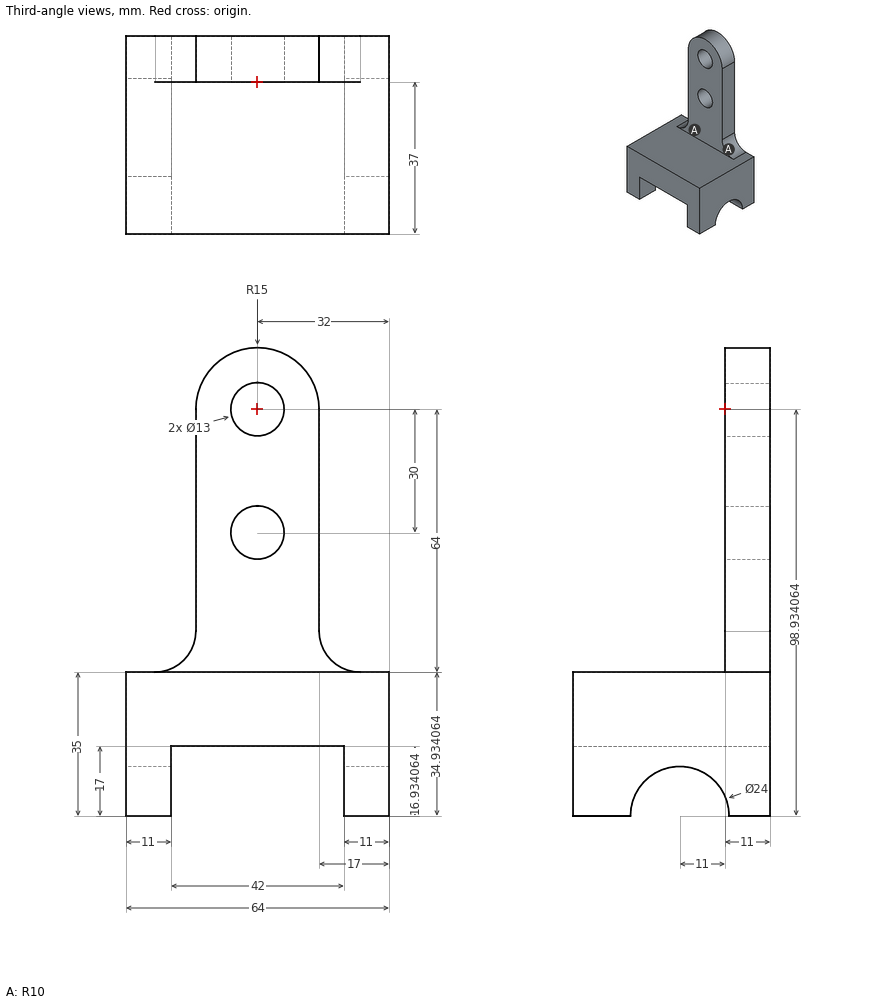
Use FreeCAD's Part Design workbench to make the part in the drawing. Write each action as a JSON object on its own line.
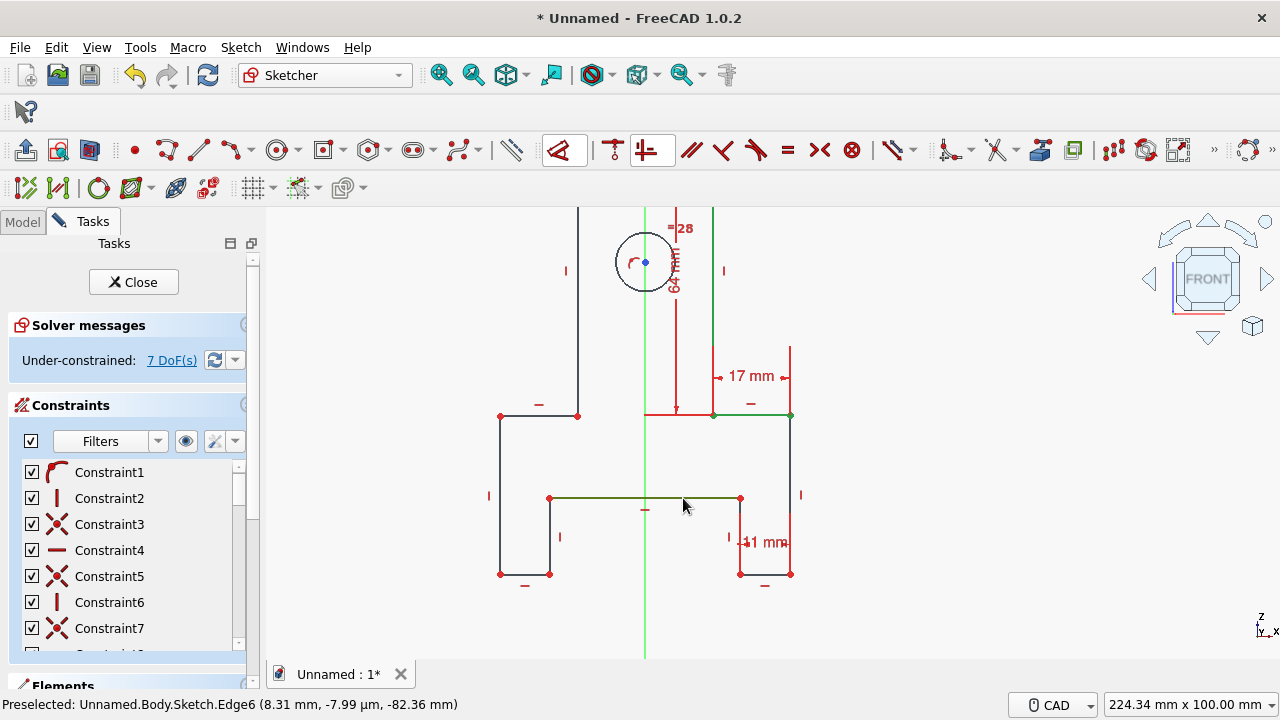
{"action": "key", "text": "l"}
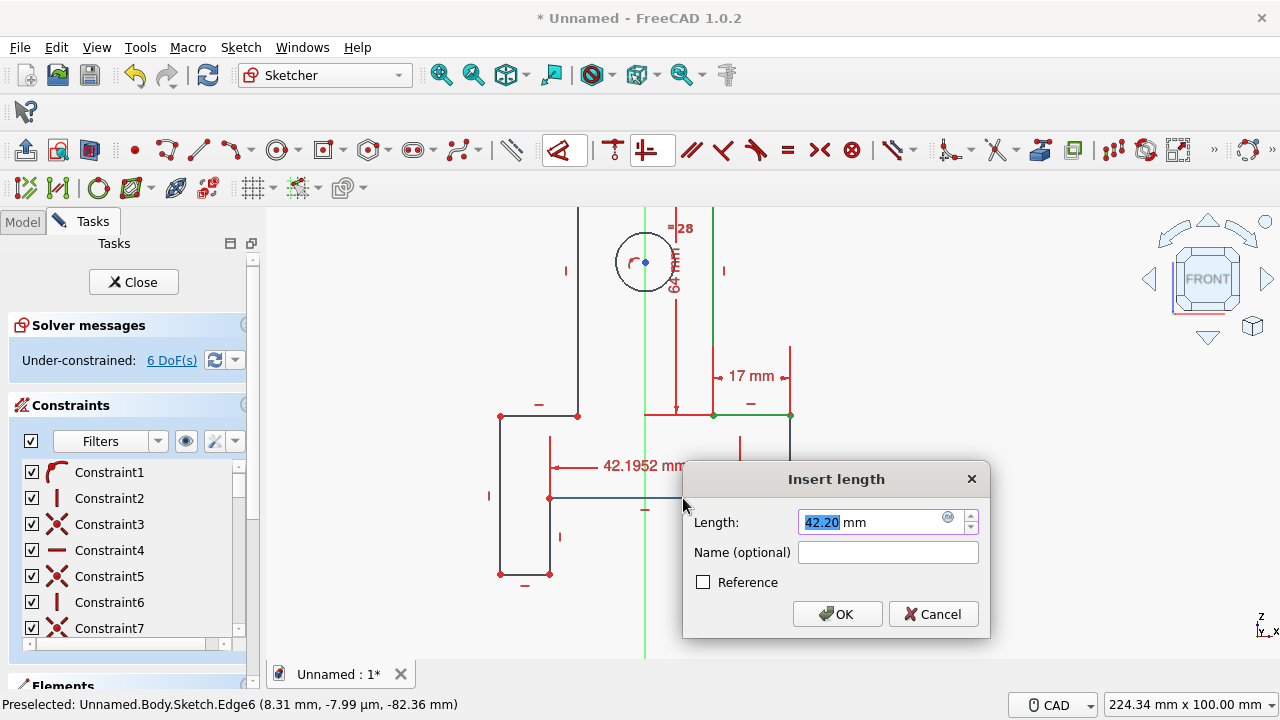
{"action": "type", "text": "42"}
{"action": "key", "text": "Return"}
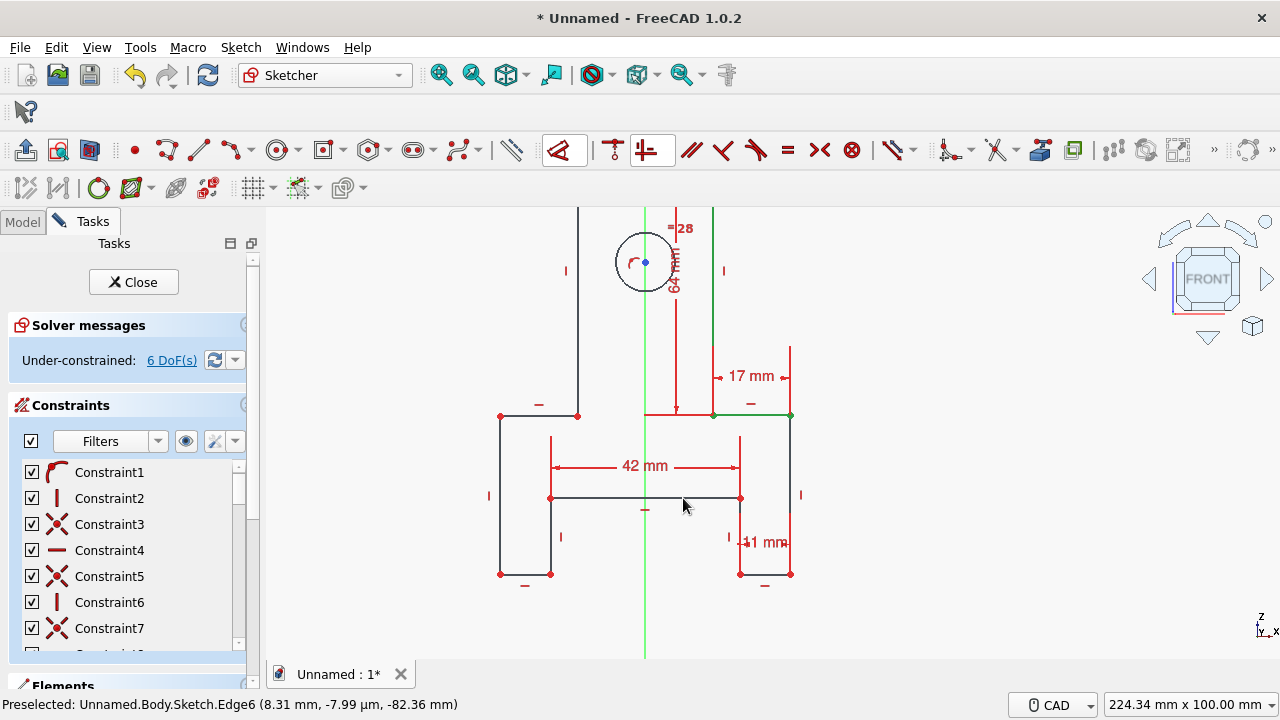
{"action": "left_click", "coordinate": [551, 521]}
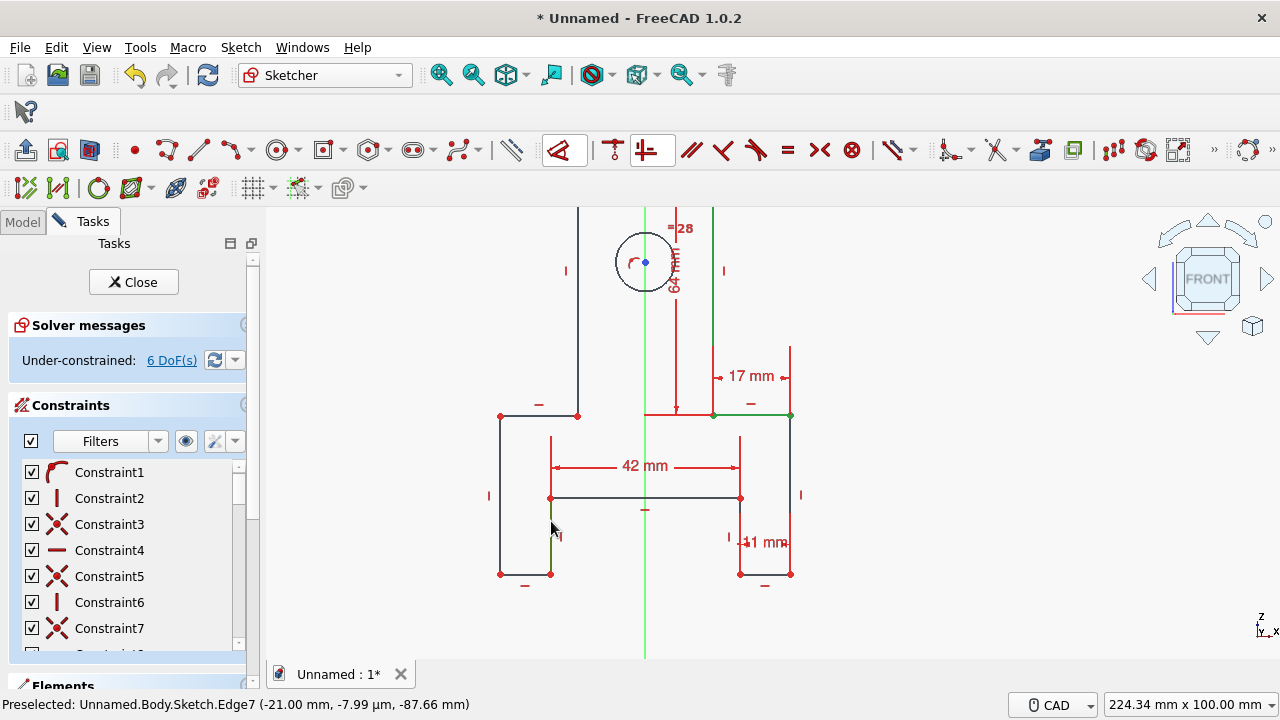
{"action": "key", "text": "i"}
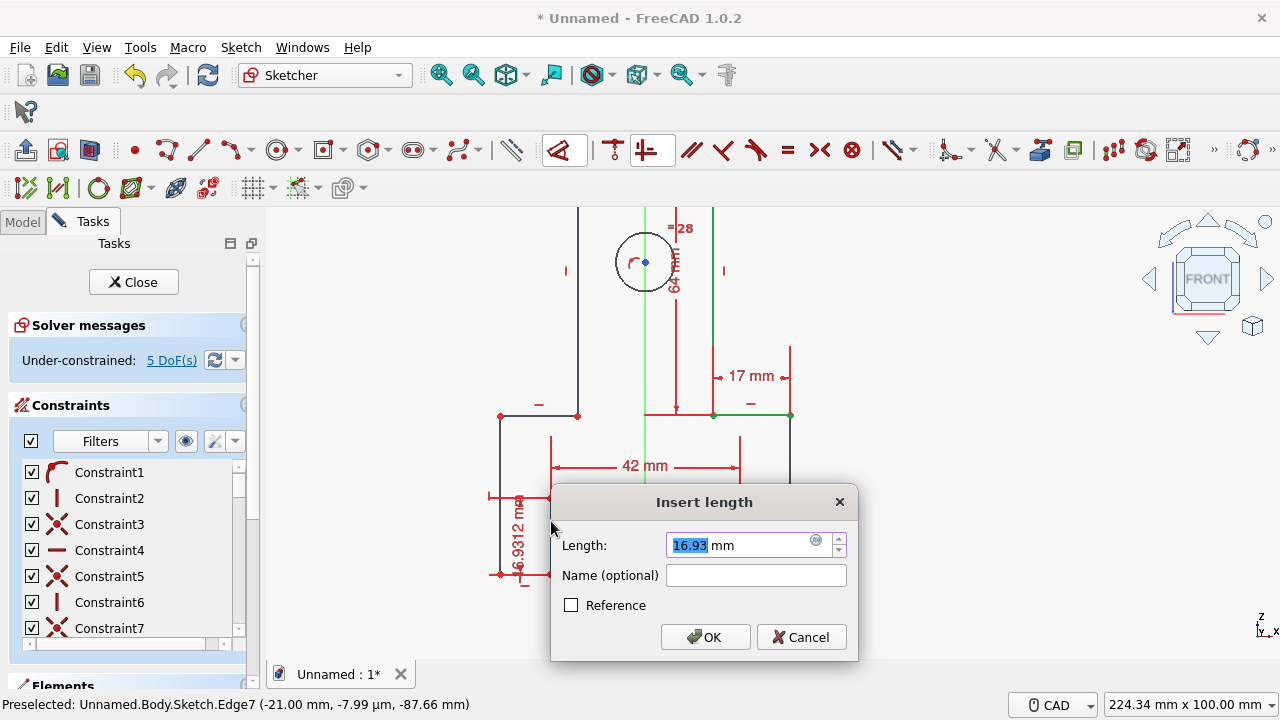
{"action": "type", "text": "17"}
{"action": "key", "text": "Return"}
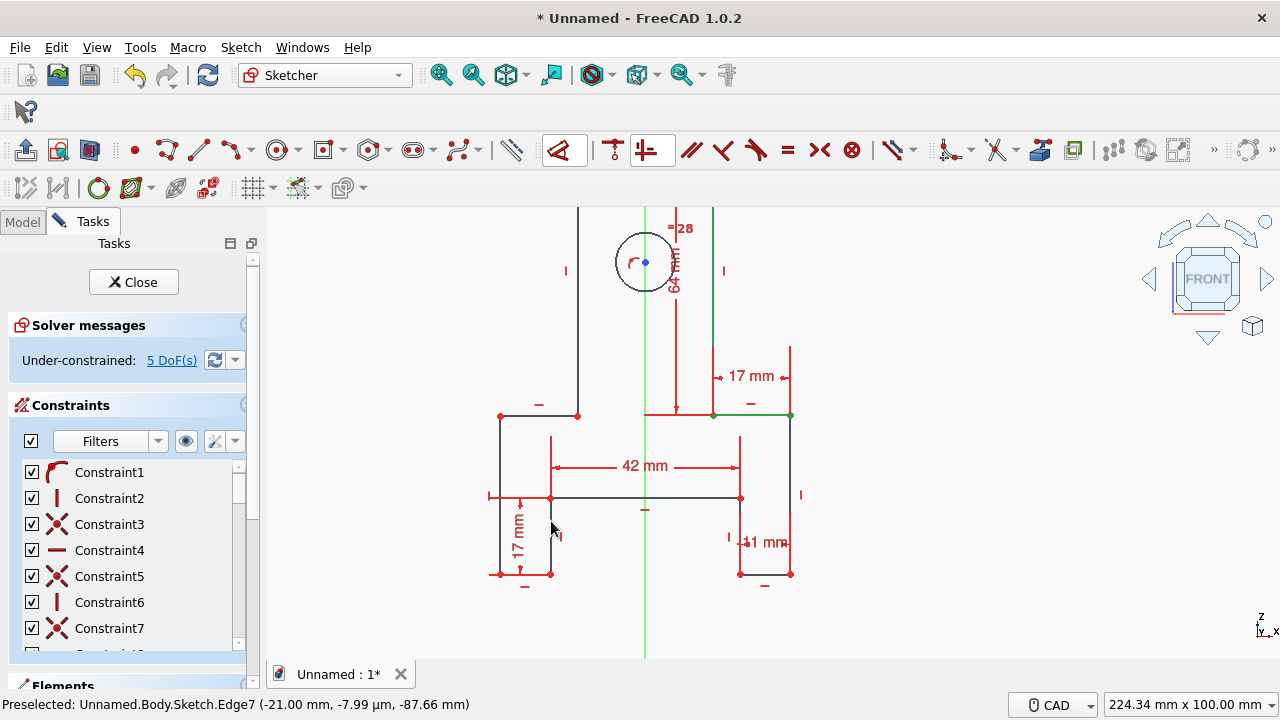
{"action": "left_click", "coordinate": [536, 575]}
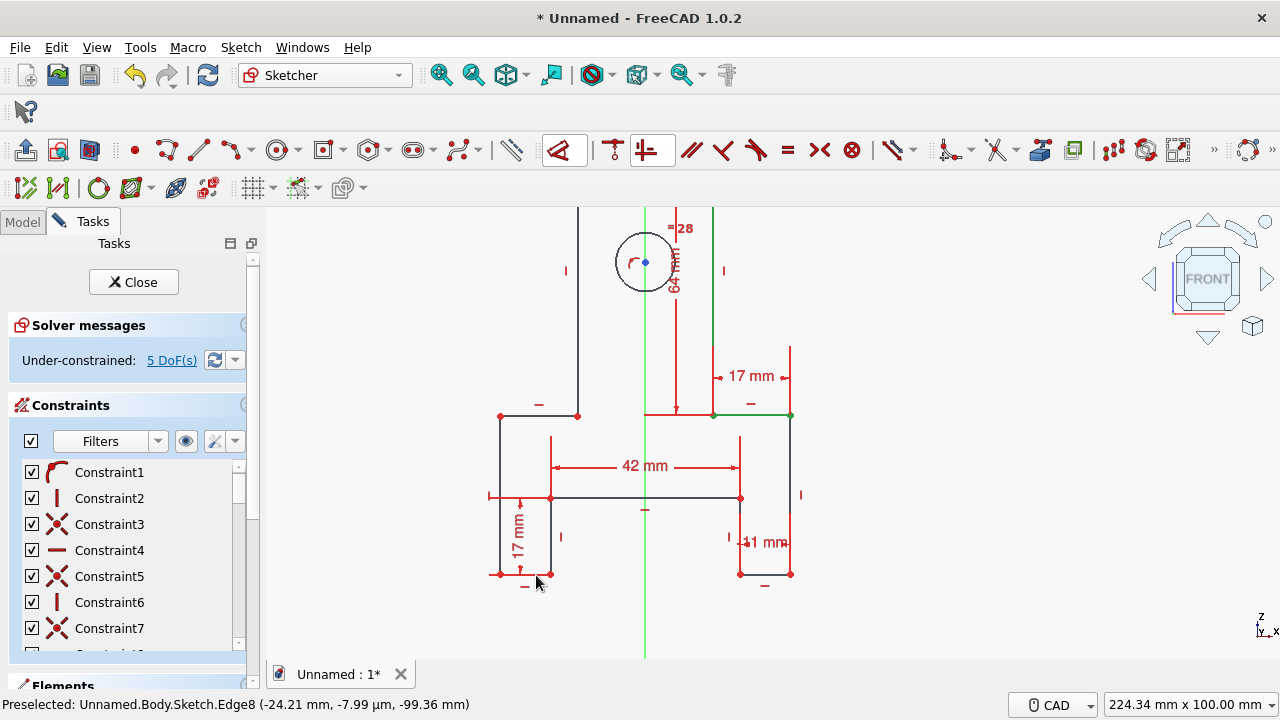
{"action": "left_click", "coordinate": [582, 150]}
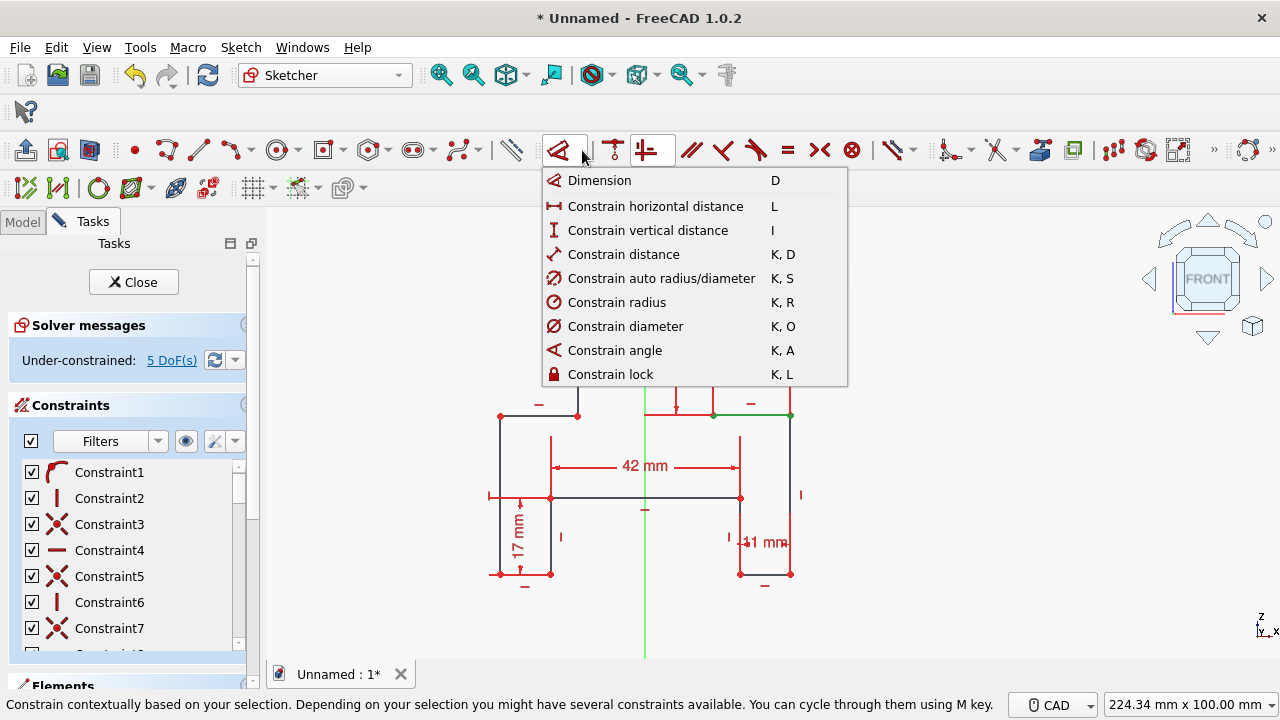
{"action": "left_click", "coordinate": [695, 206]}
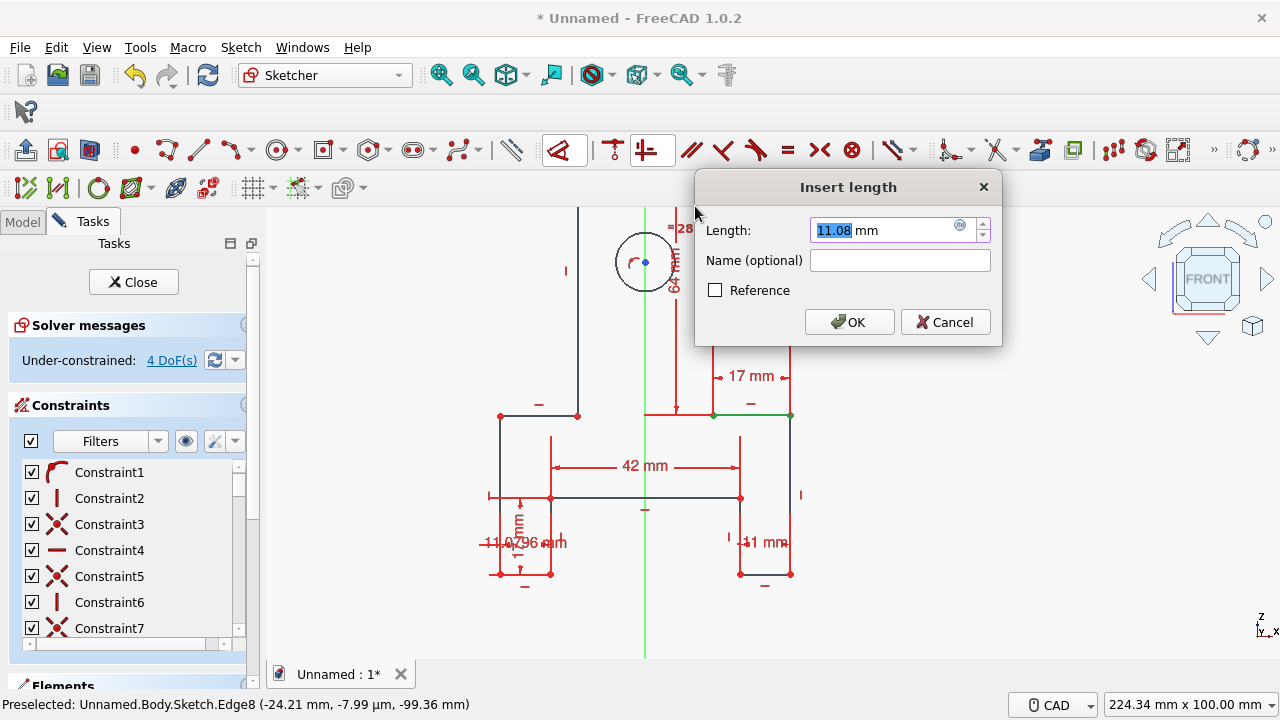
{"action": "type", "text": "11"}
{"action": "key", "text": "Return"}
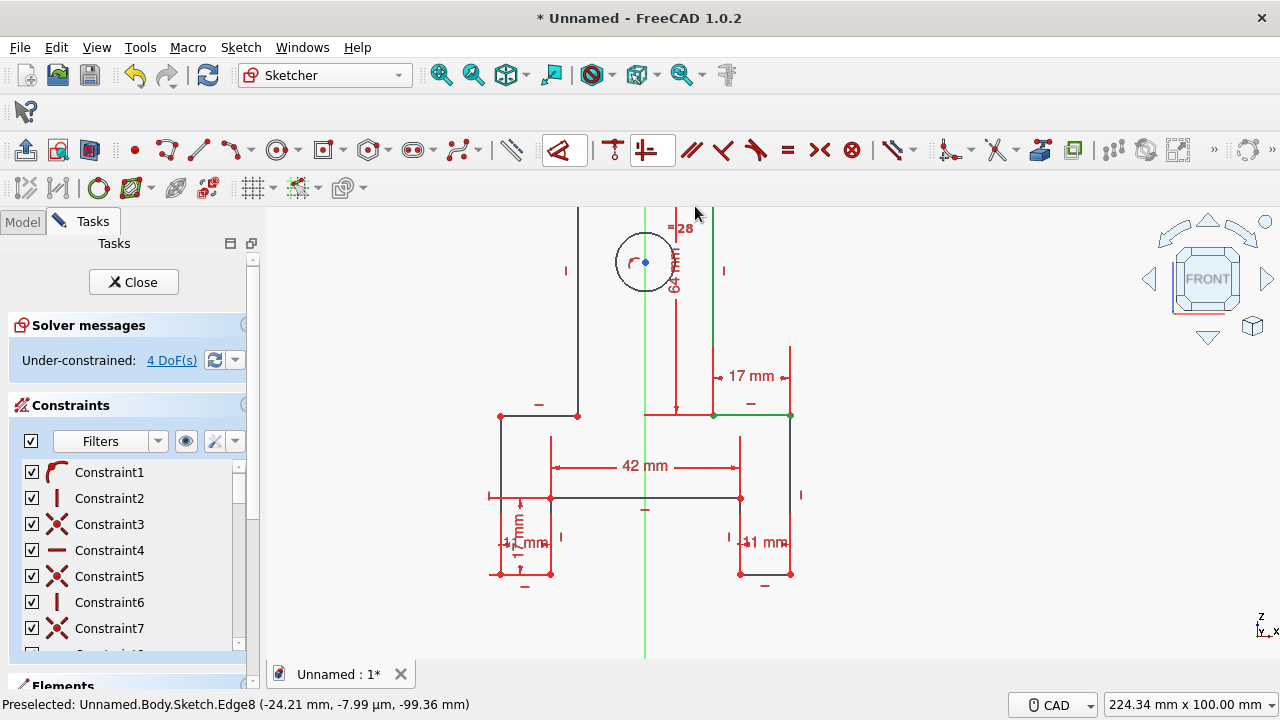
{"action": "left_click", "coordinate": [501, 527]}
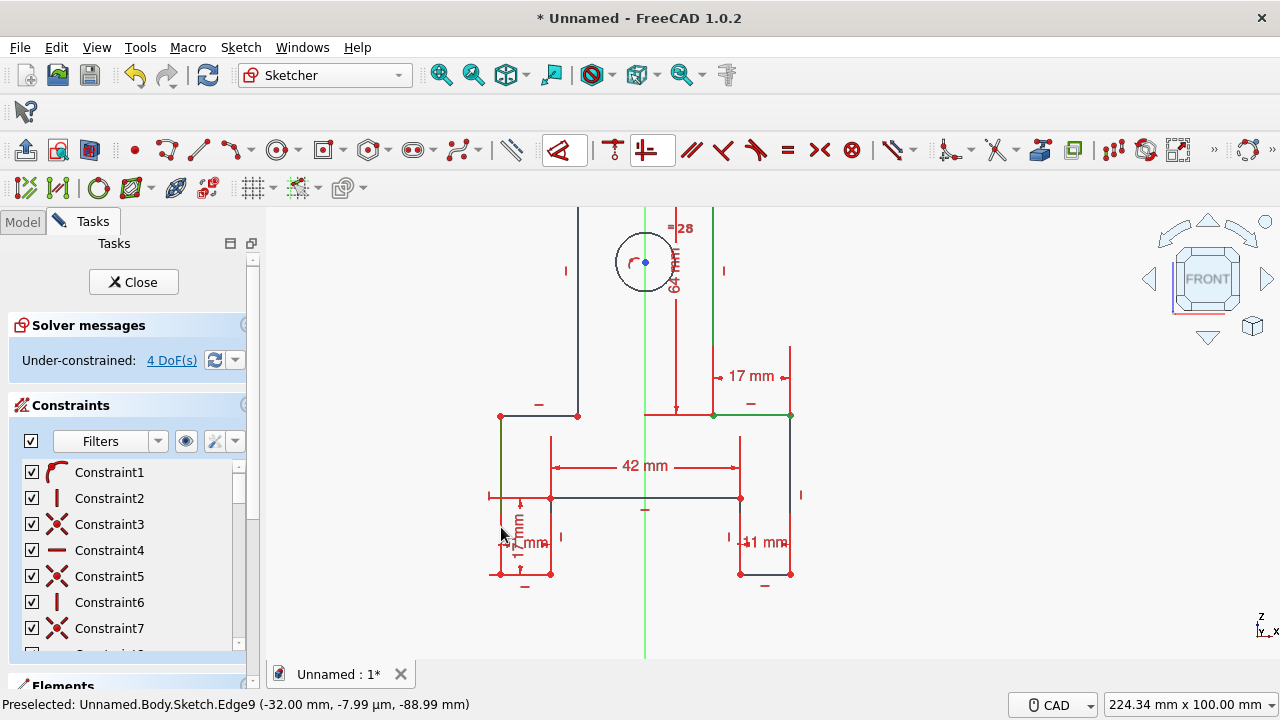
{"action": "left_click", "coordinate": [582, 150]}